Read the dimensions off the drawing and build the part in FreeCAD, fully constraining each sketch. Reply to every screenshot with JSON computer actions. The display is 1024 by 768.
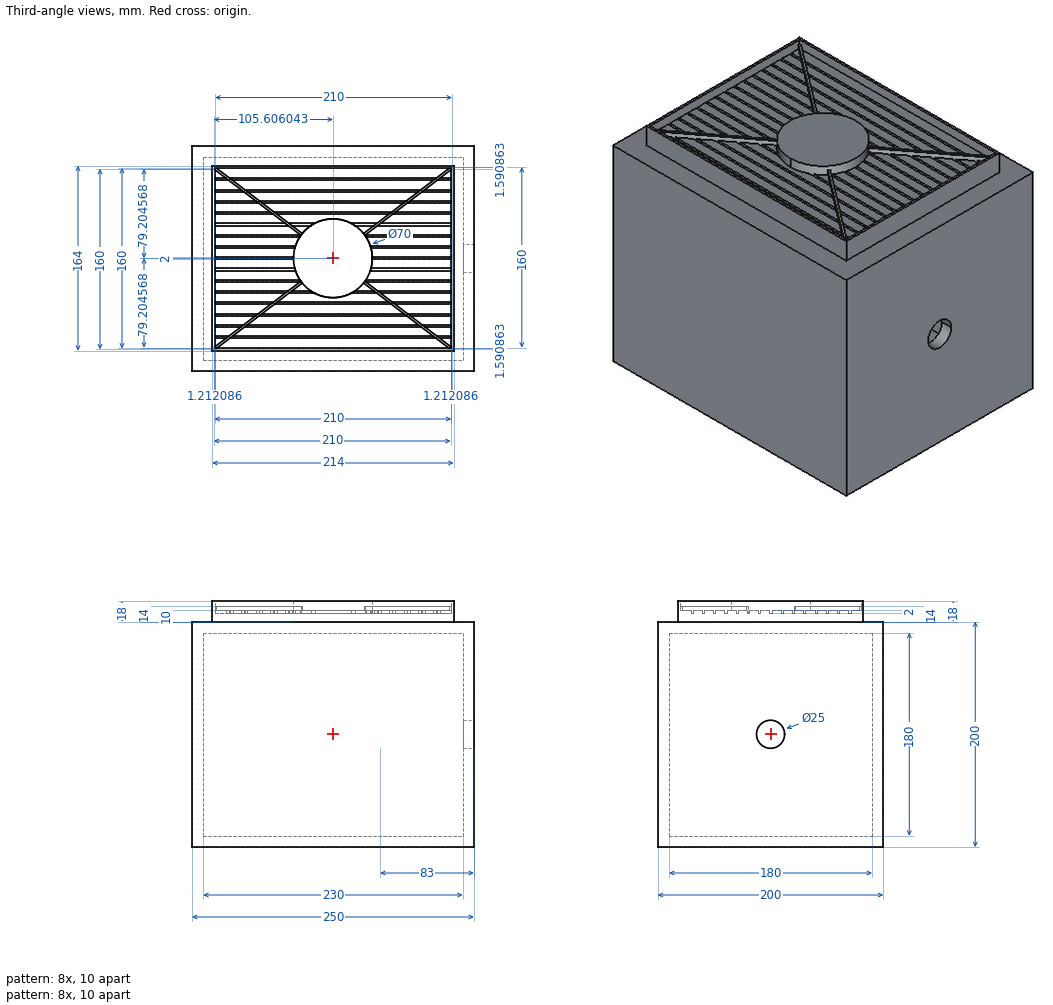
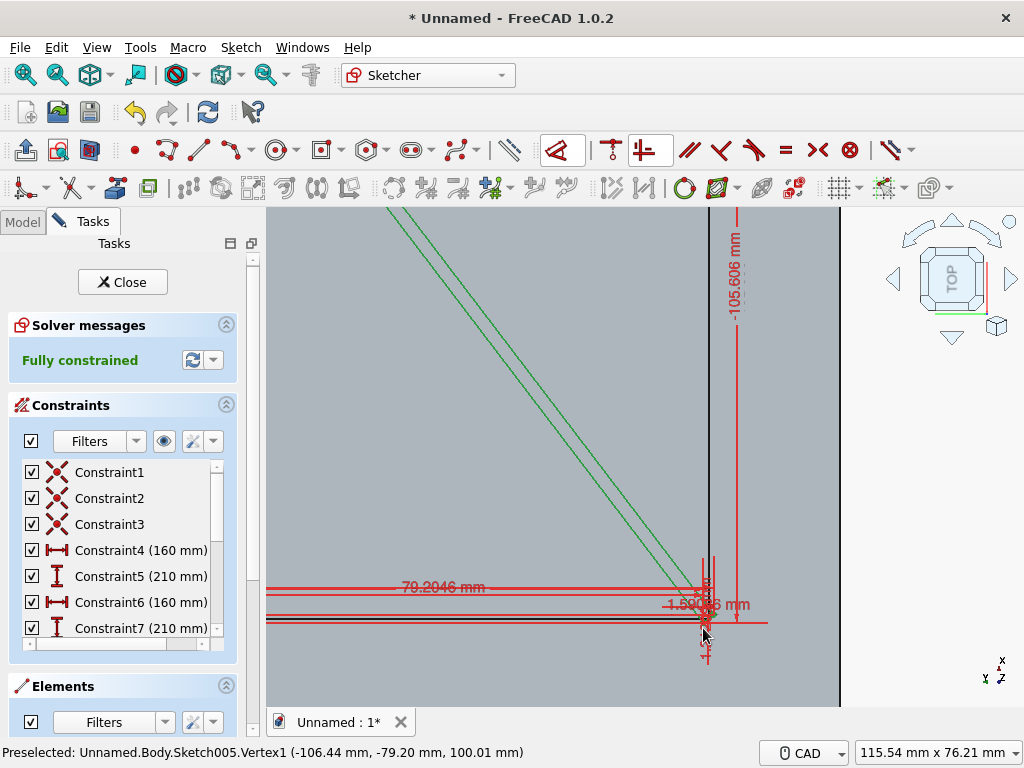
{"action": "left_click", "coordinate": [123, 282]}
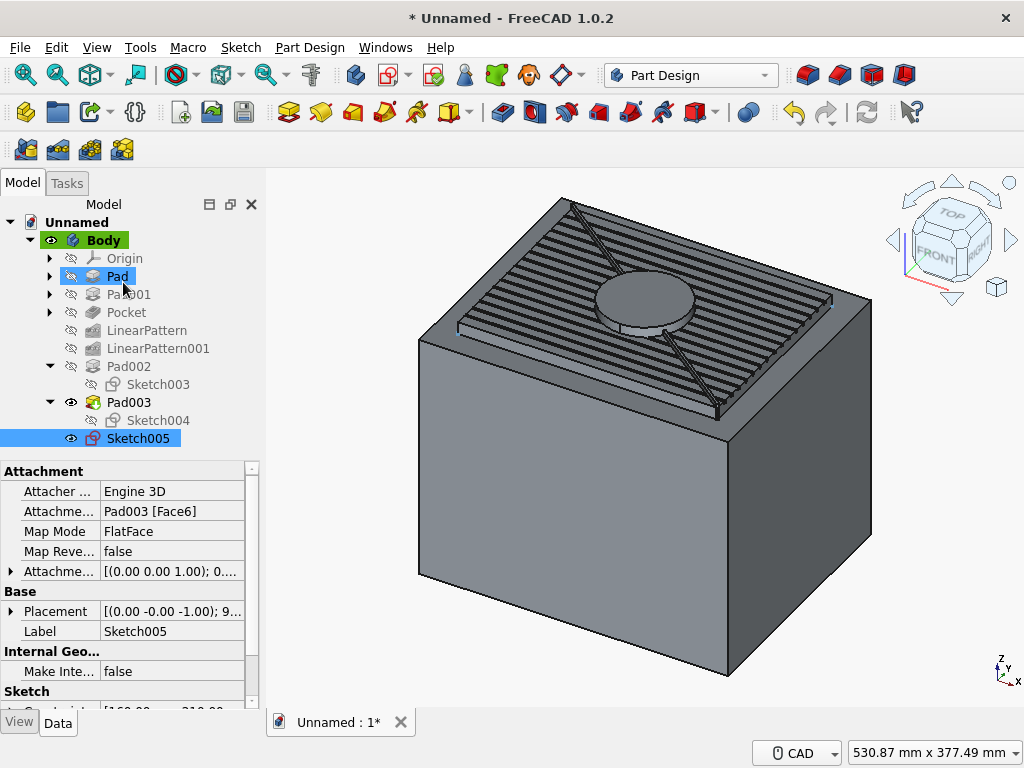
{"action": "left_click", "coordinate": [290, 112]}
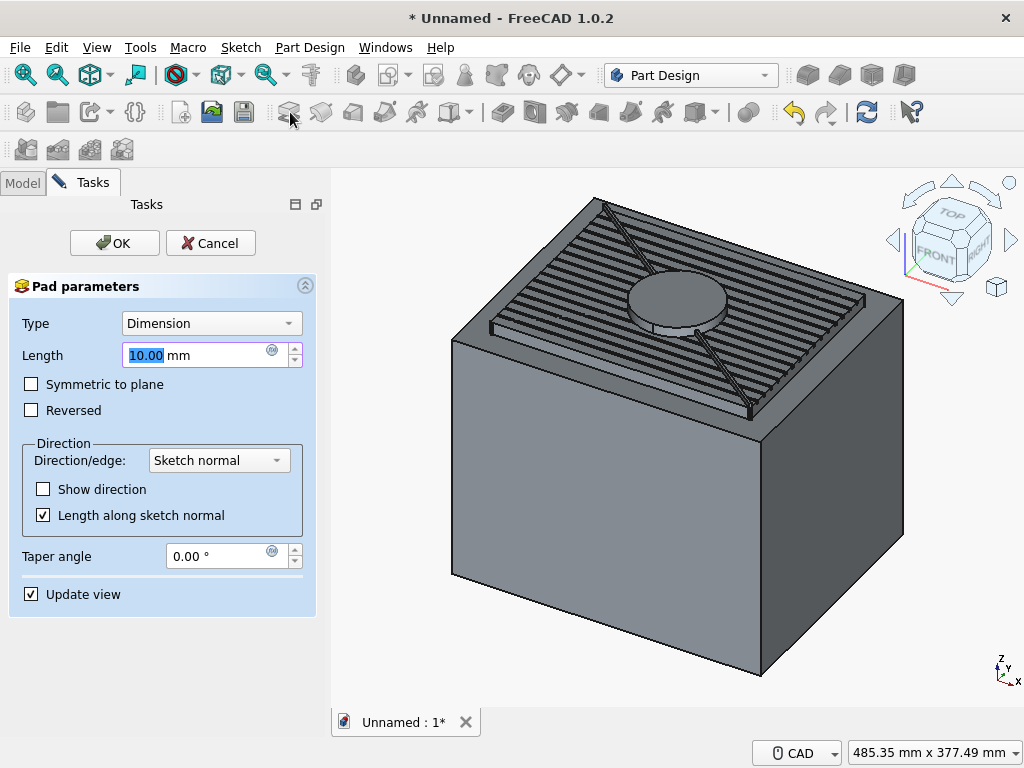
{"action": "type", "text": "14"}
{"action": "key", "text": "Tab"}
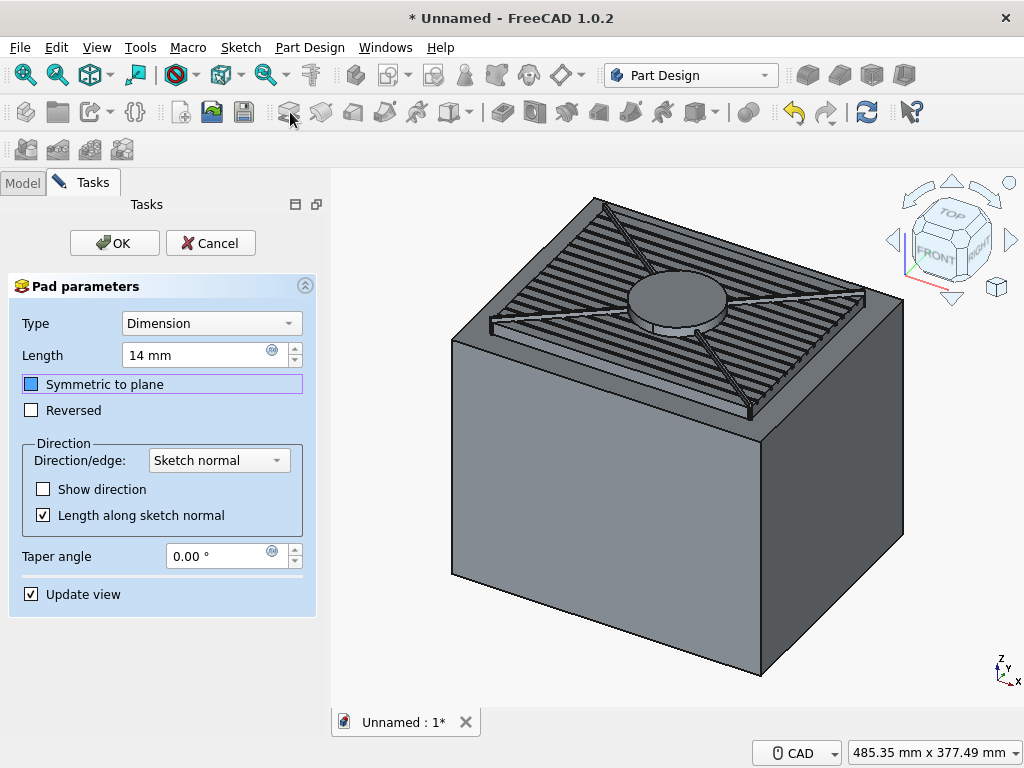
{"action": "left_click", "coordinate": [115, 243]}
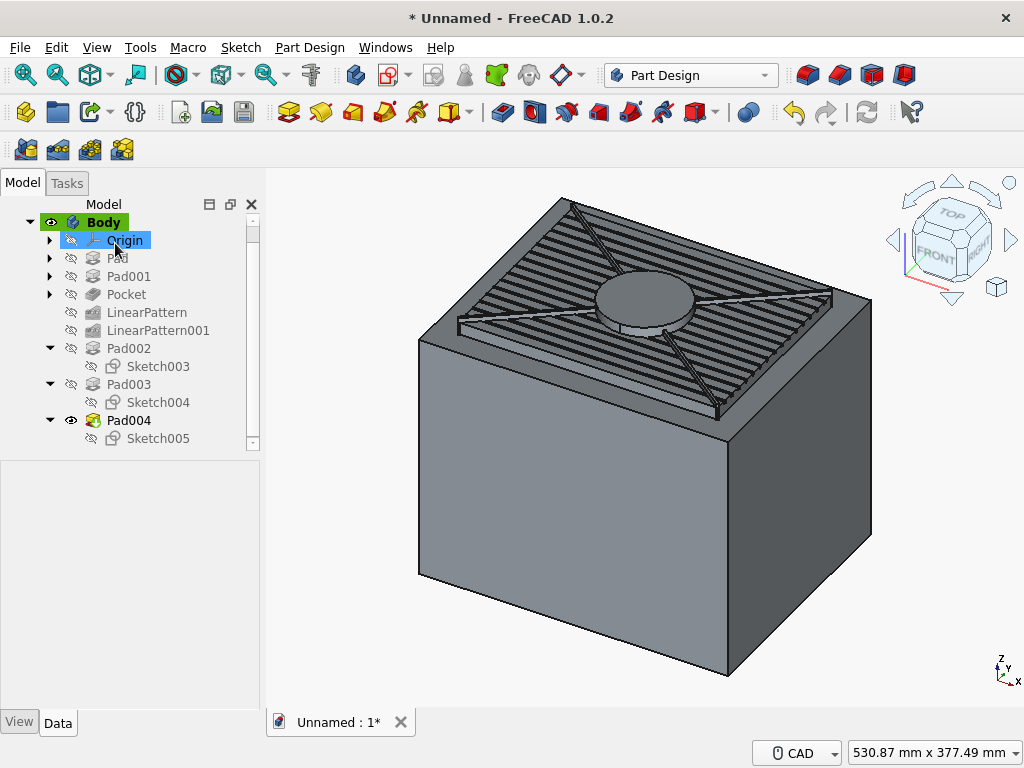
{"action": "left_click", "coordinate": [672, 409]}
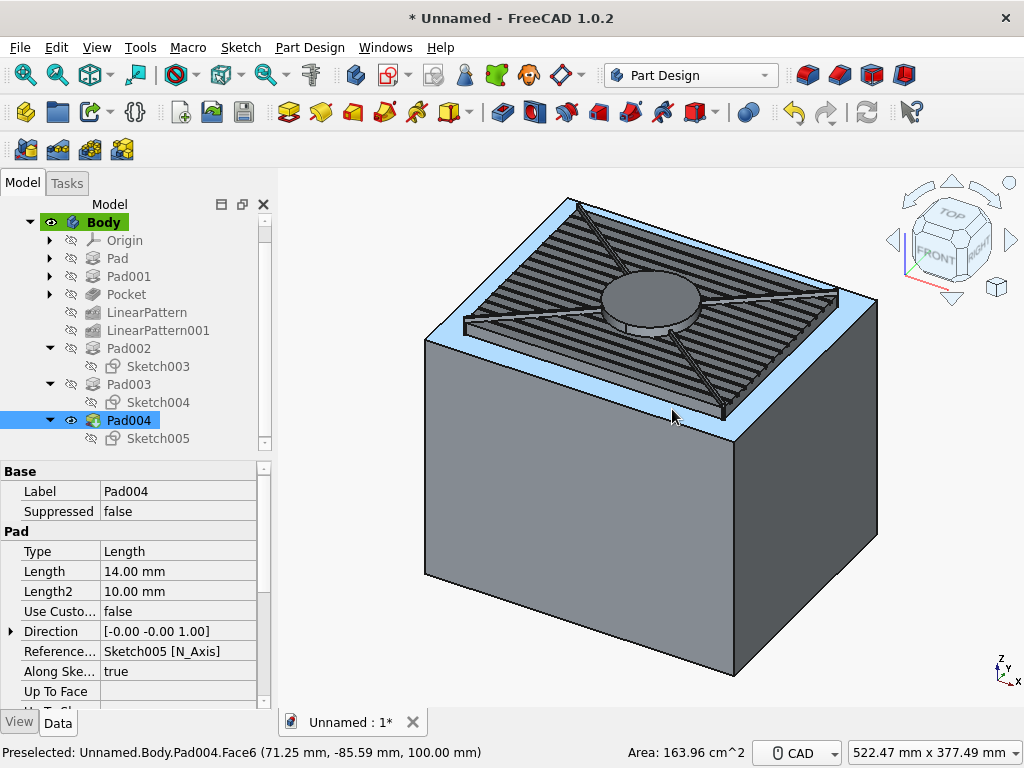
{"action": "left_click", "coordinate": [388, 76]}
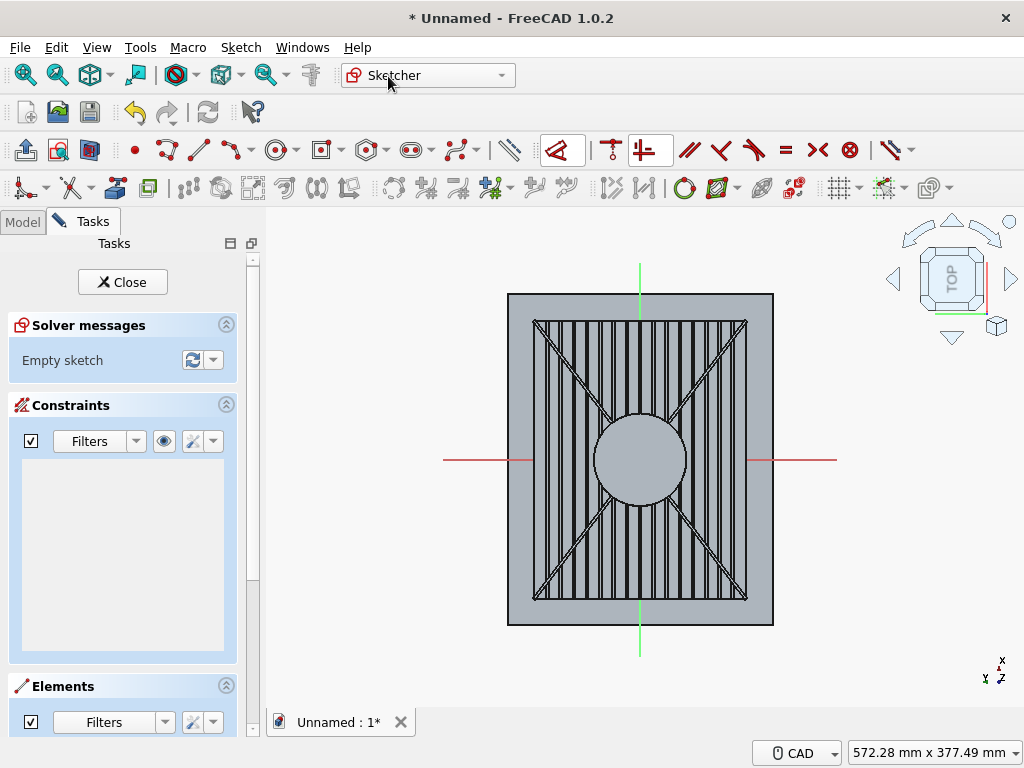
{"action": "left_click", "coordinate": [322, 150]}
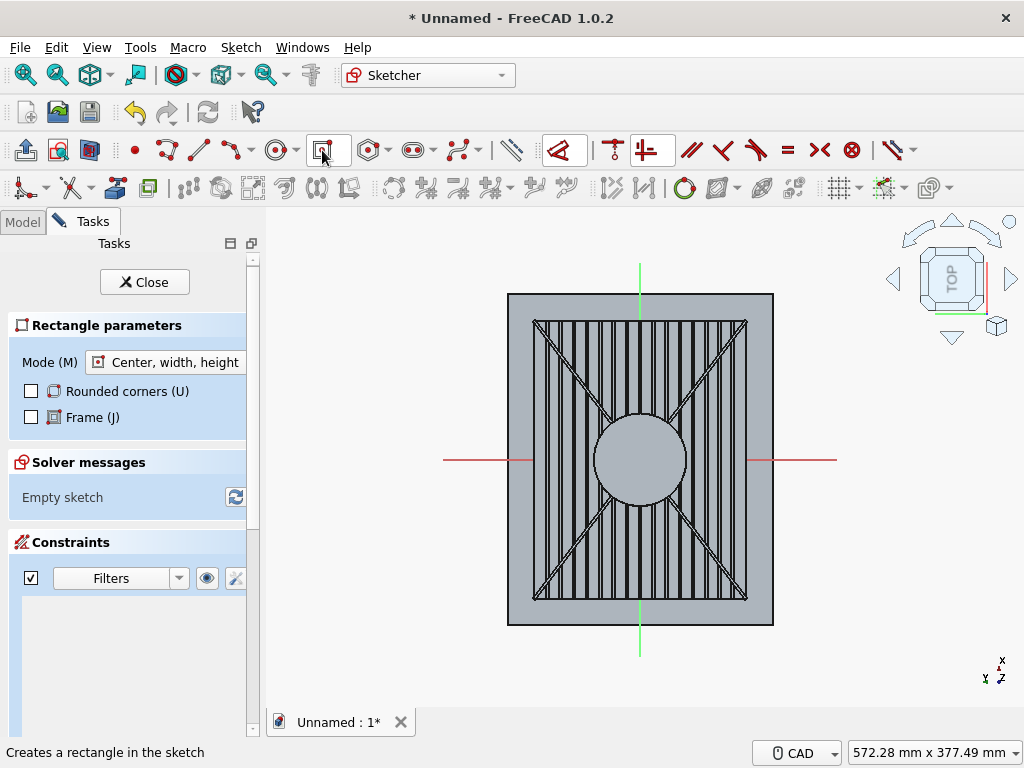
{"action": "left_click", "coordinate": [640, 460]}
{"action": "left_click", "coordinate": [749, 318]}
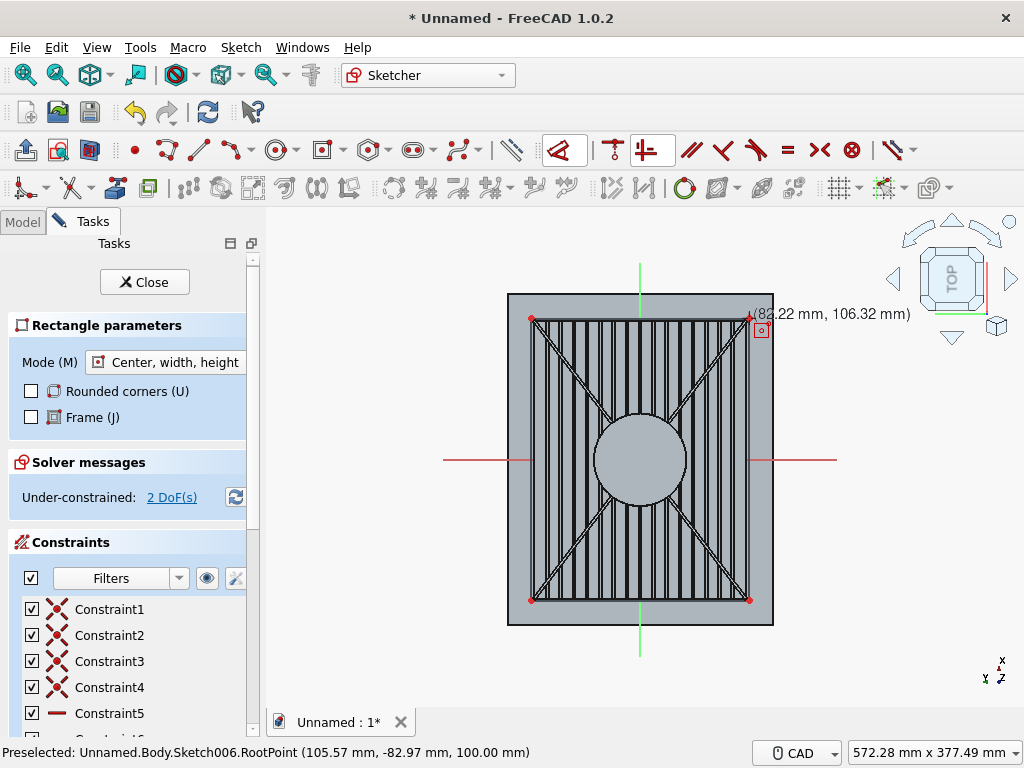
{"action": "left_click", "coordinate": [640, 460]}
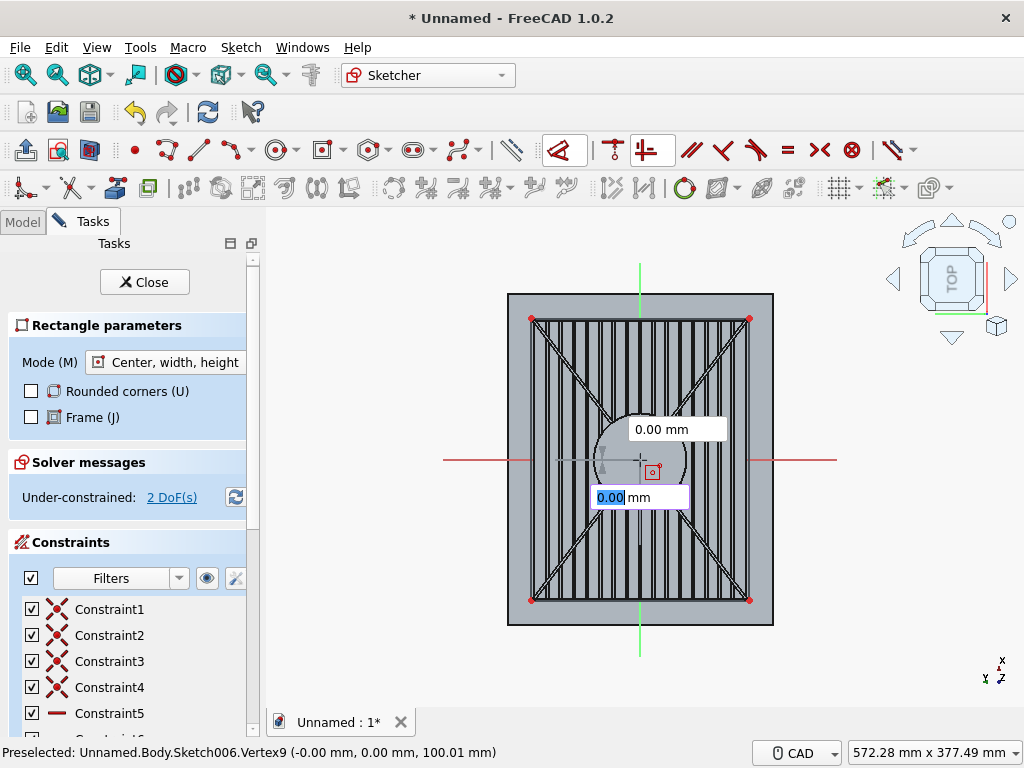
{"action": "scroll", "coordinate": [746, 321], "scroll_direction": "up", "scroll_amount": 9}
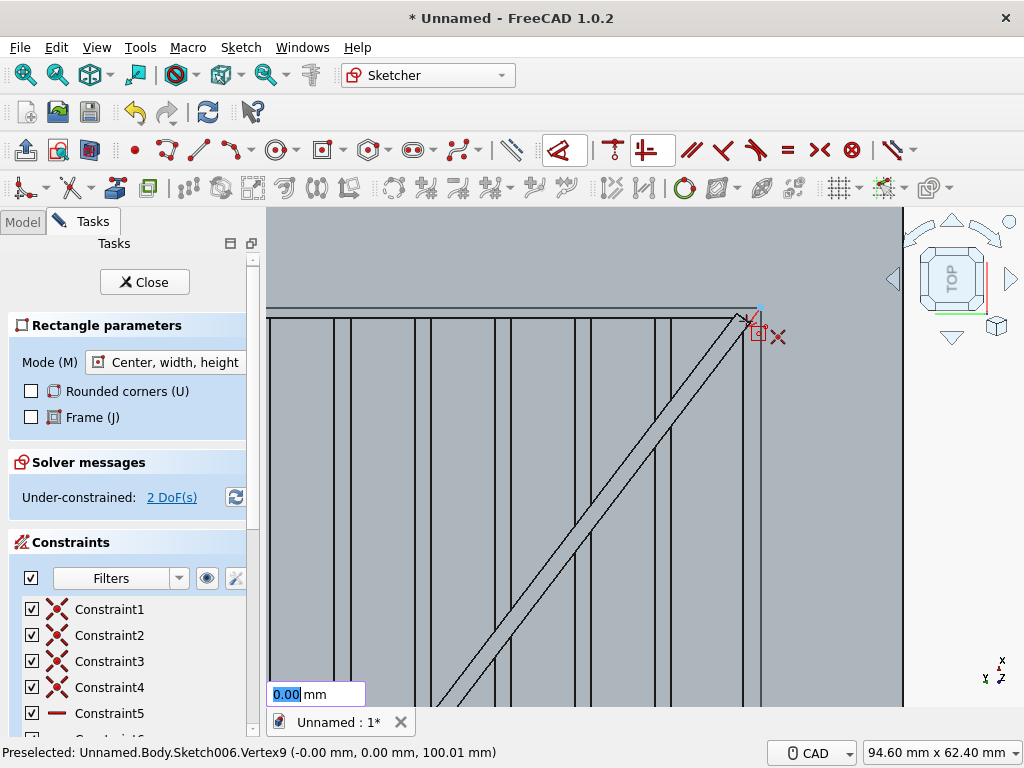
{"action": "left_click", "coordinate": [743, 318]}
{"action": "key", "text": "Escape"}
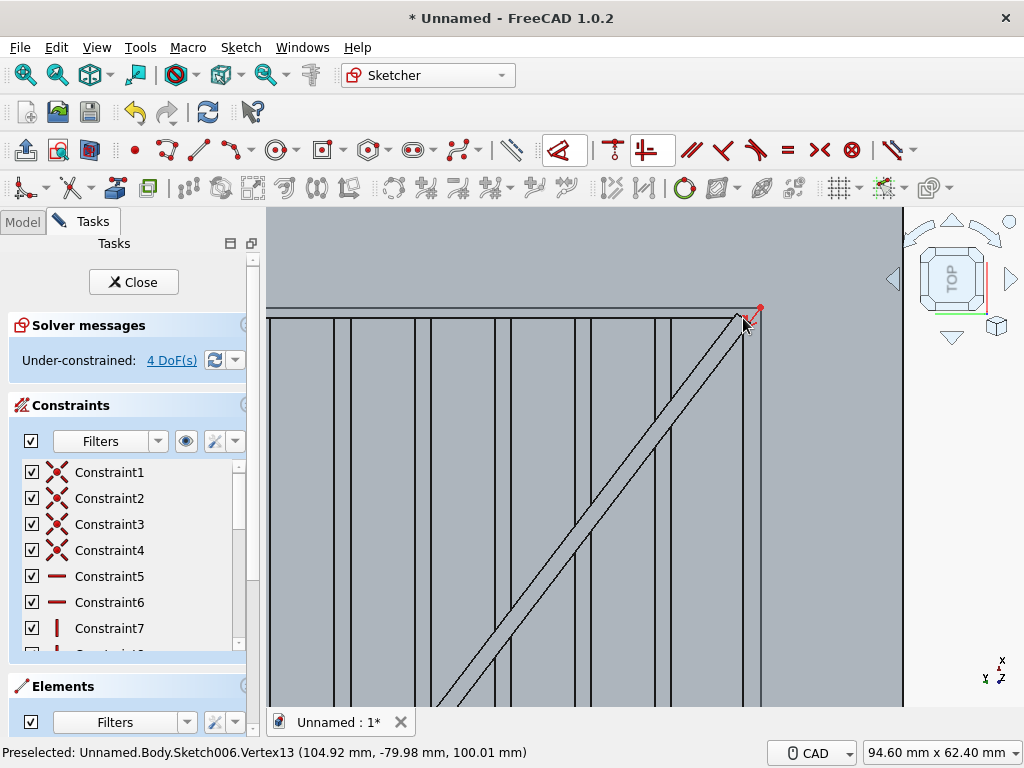
{"action": "scroll", "coordinate": [697, 279], "scroll_direction": "down", "scroll_amount": 8}